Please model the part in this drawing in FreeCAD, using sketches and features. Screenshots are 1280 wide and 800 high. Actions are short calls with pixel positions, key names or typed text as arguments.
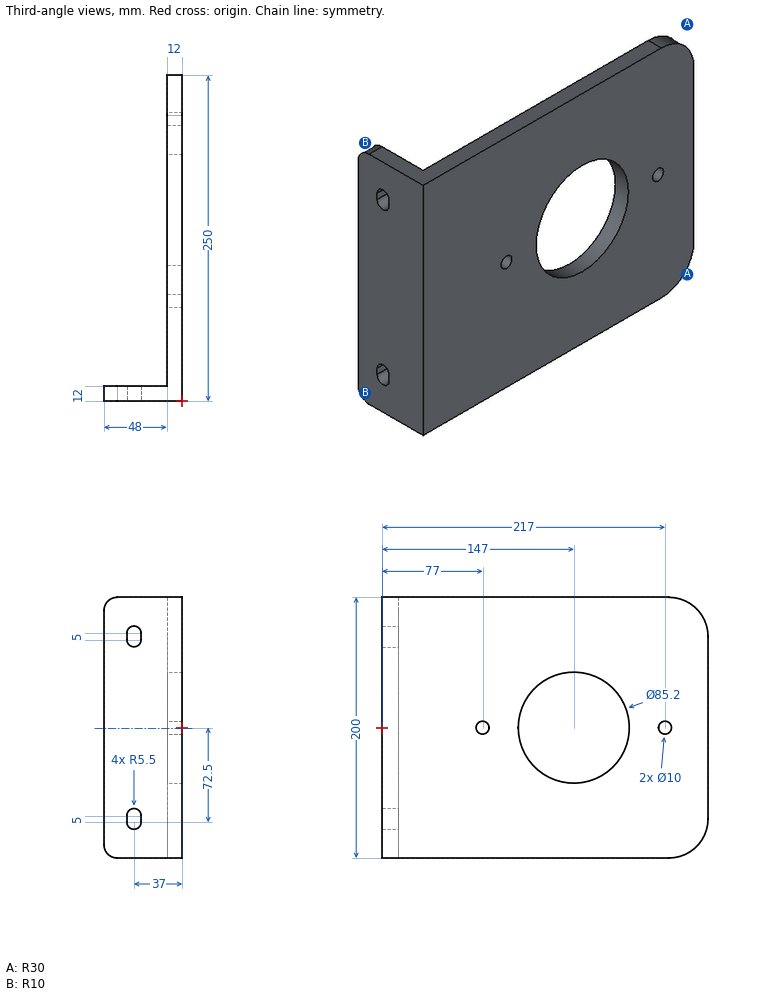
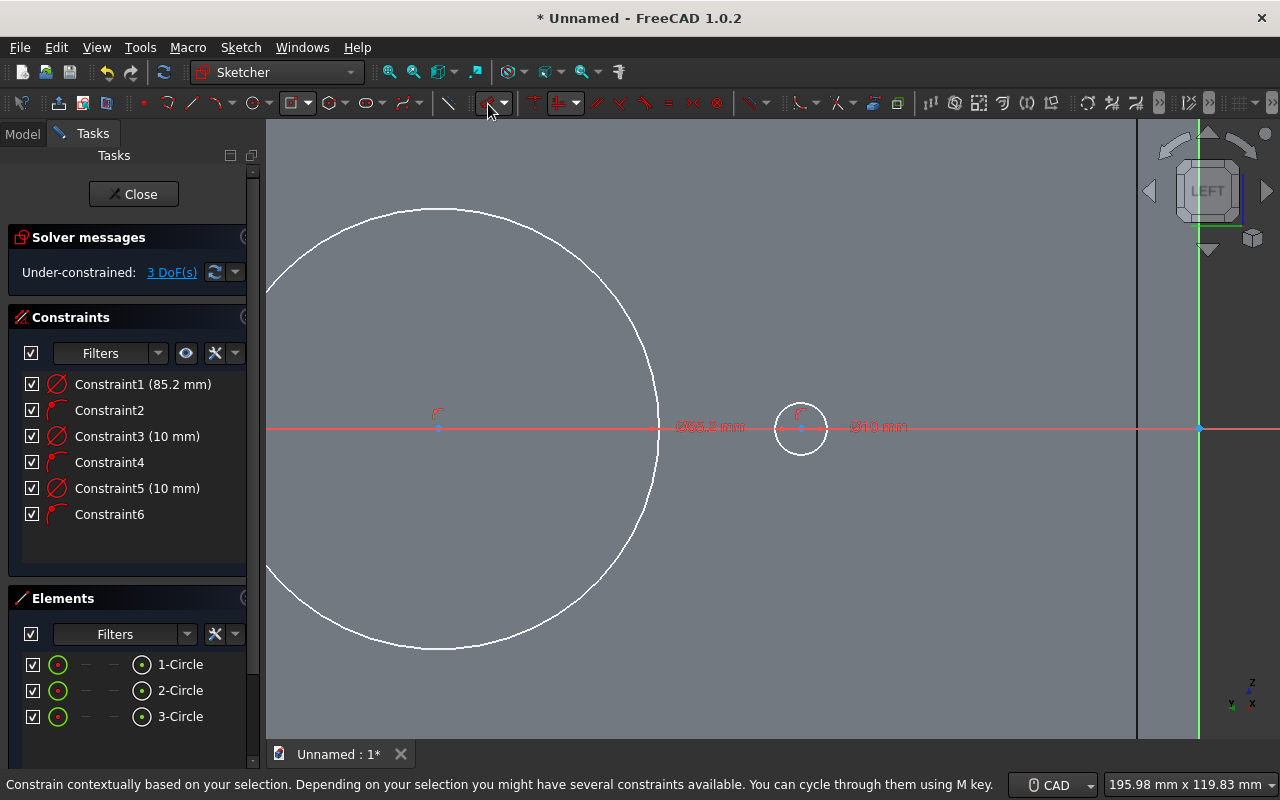
click(801, 429)
click(958, 463)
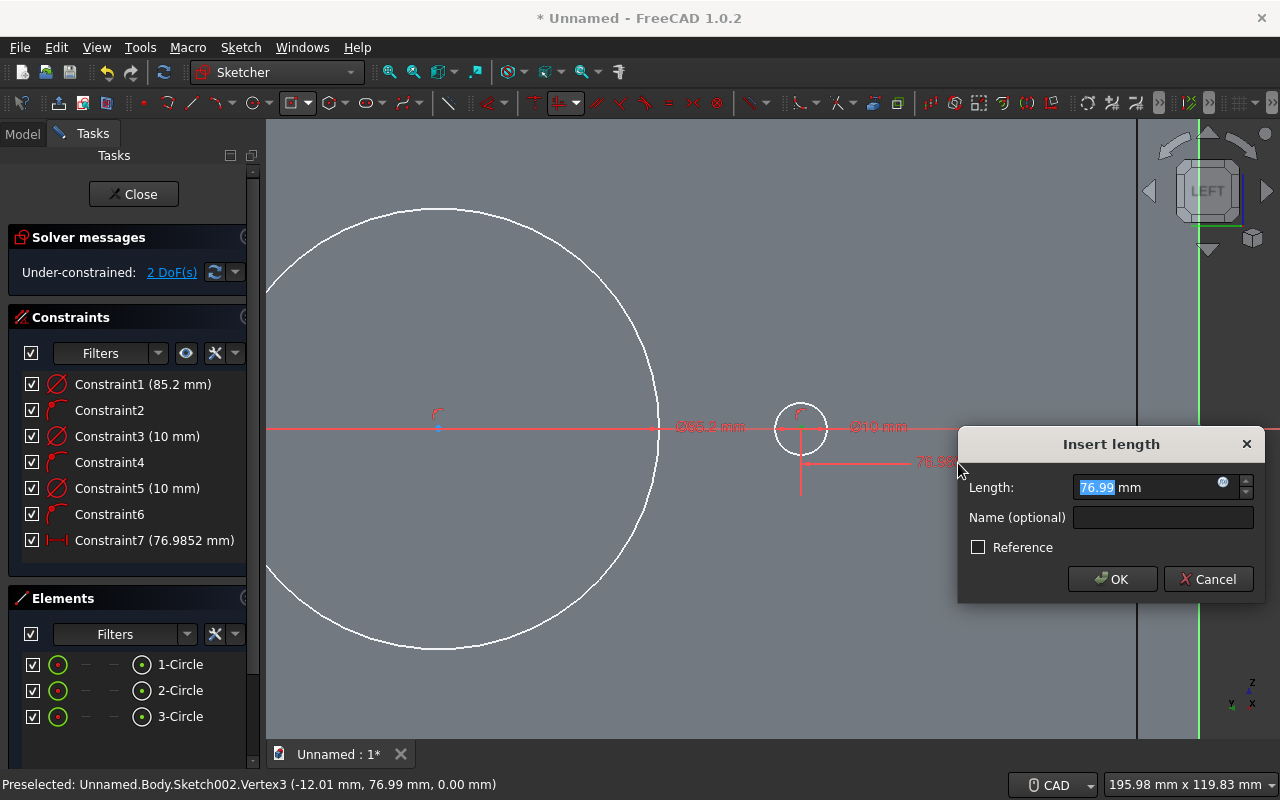
text(77)
key(Return)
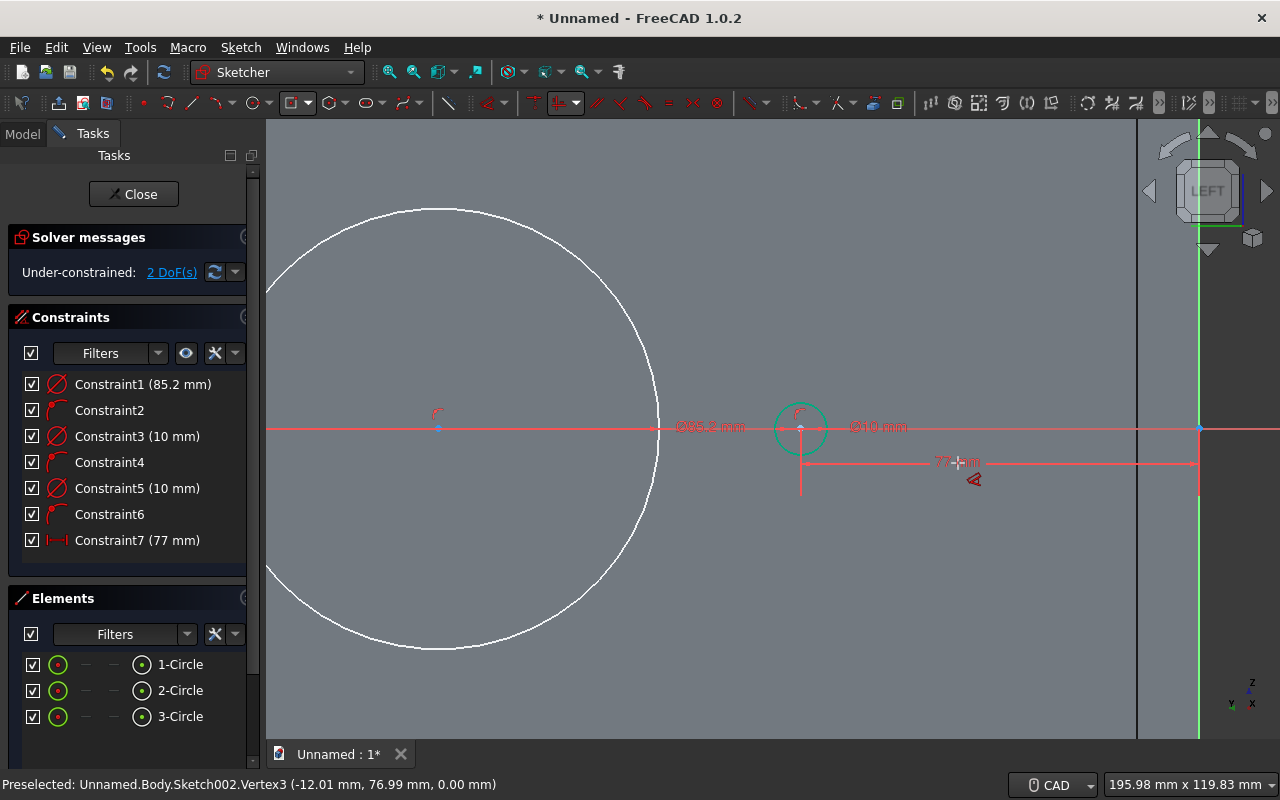
click(439, 429)
click(777, 463)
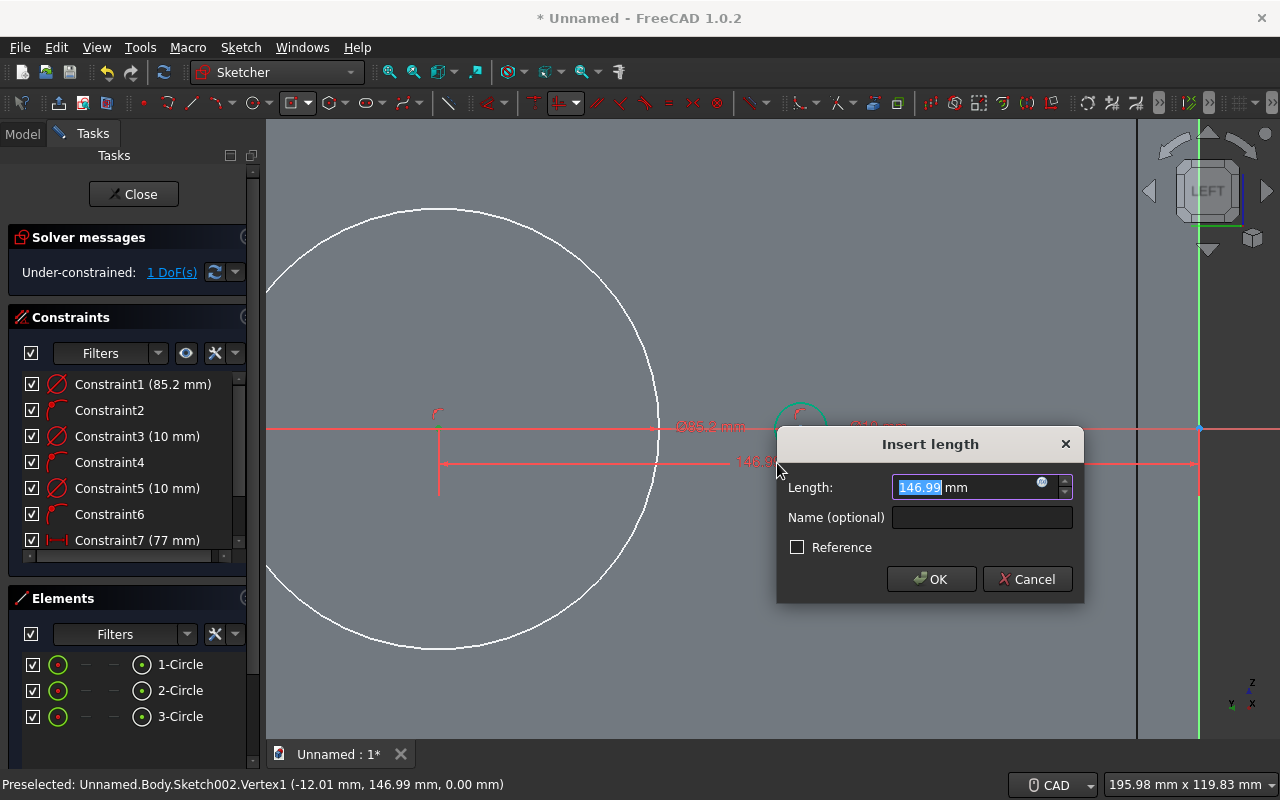
text(147)
key(Return)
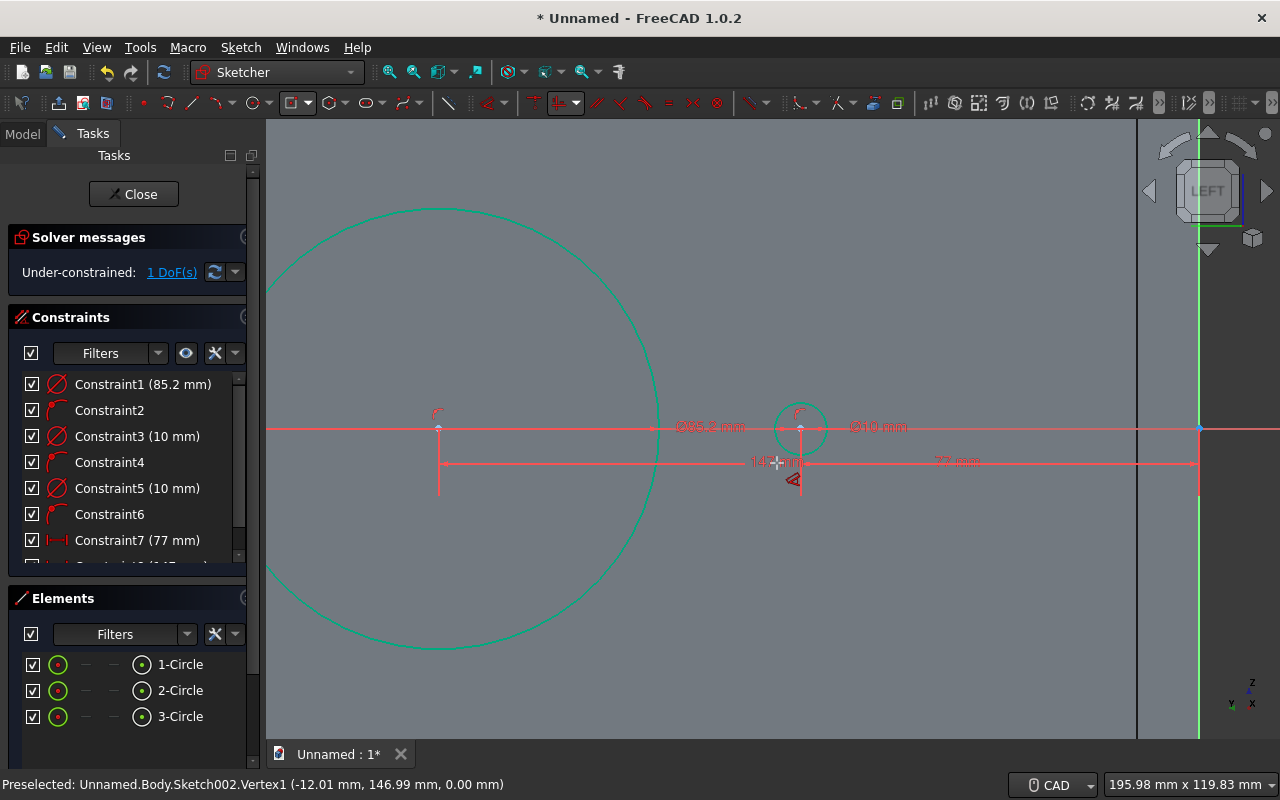
scroll(801, 429, down, 3)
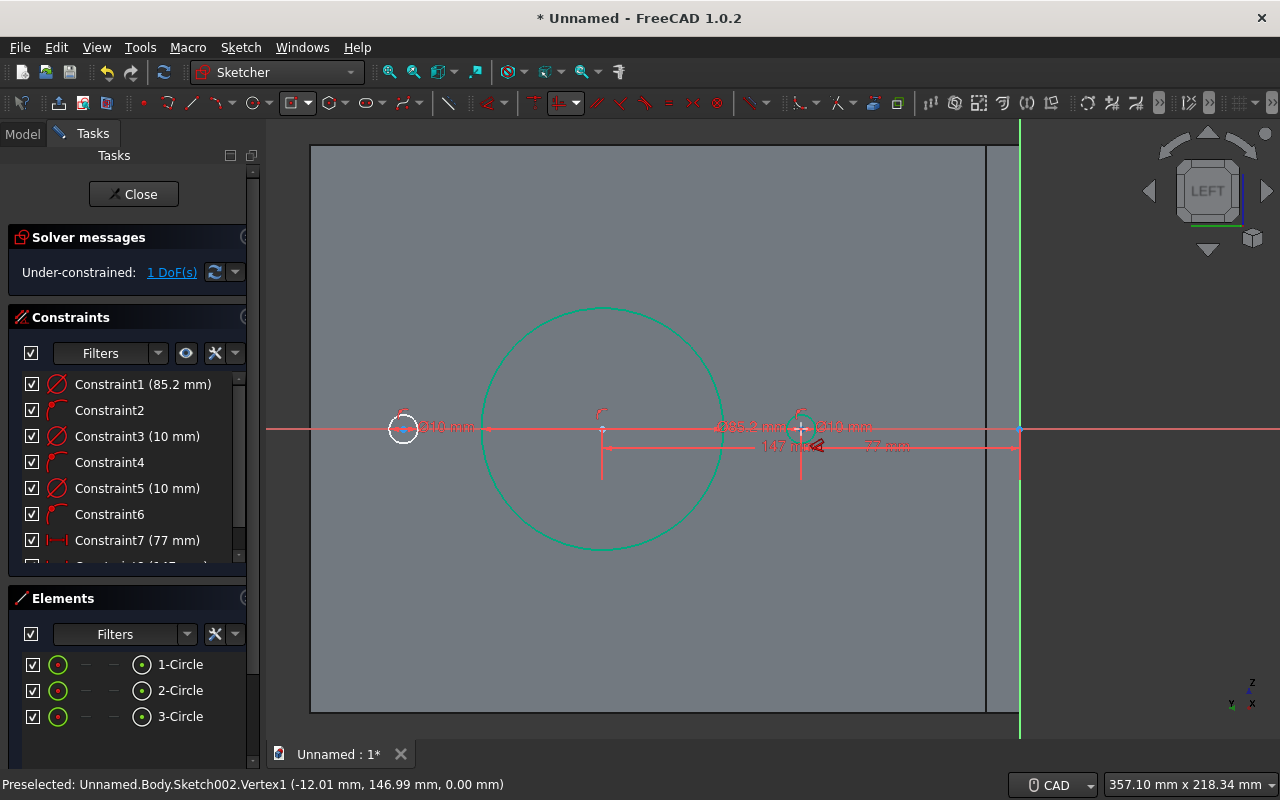
click(404, 429)
click(570, 463)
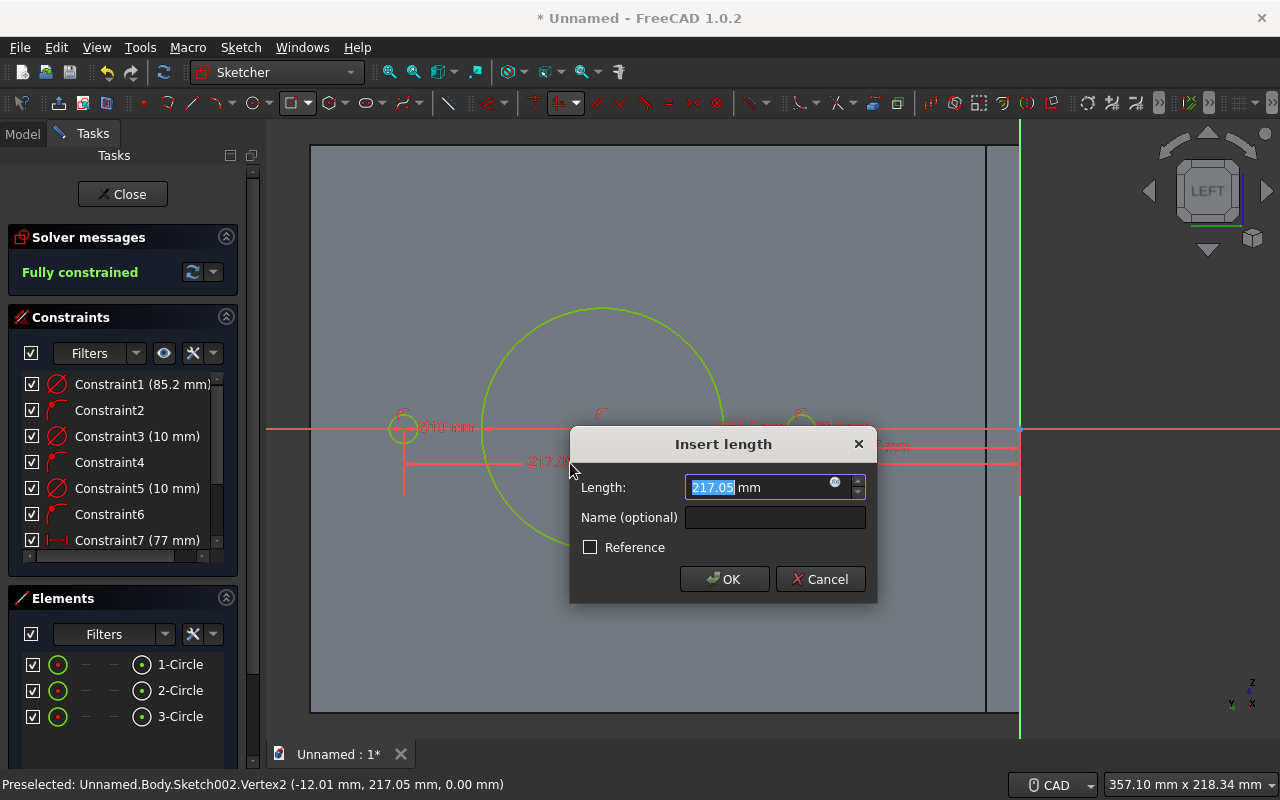
text(217)
key(Return)
key(Escape)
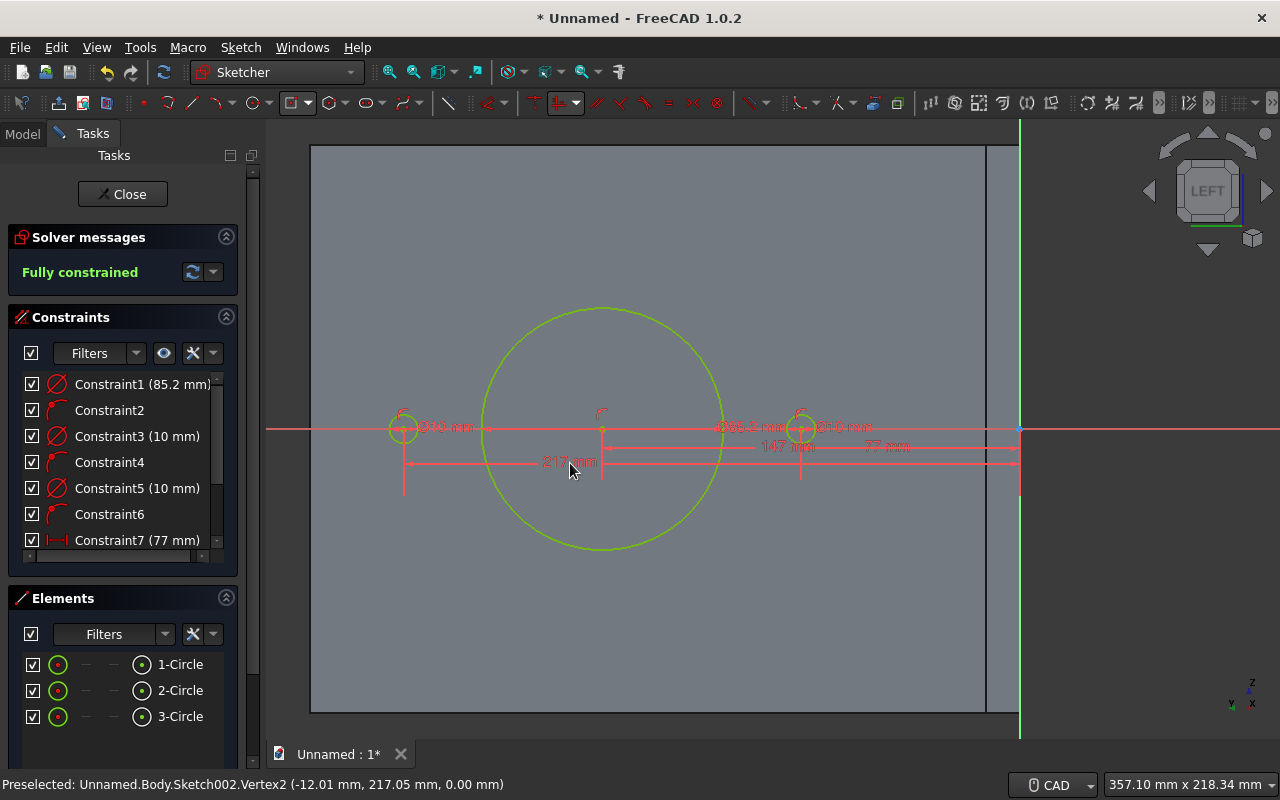
click(123, 194)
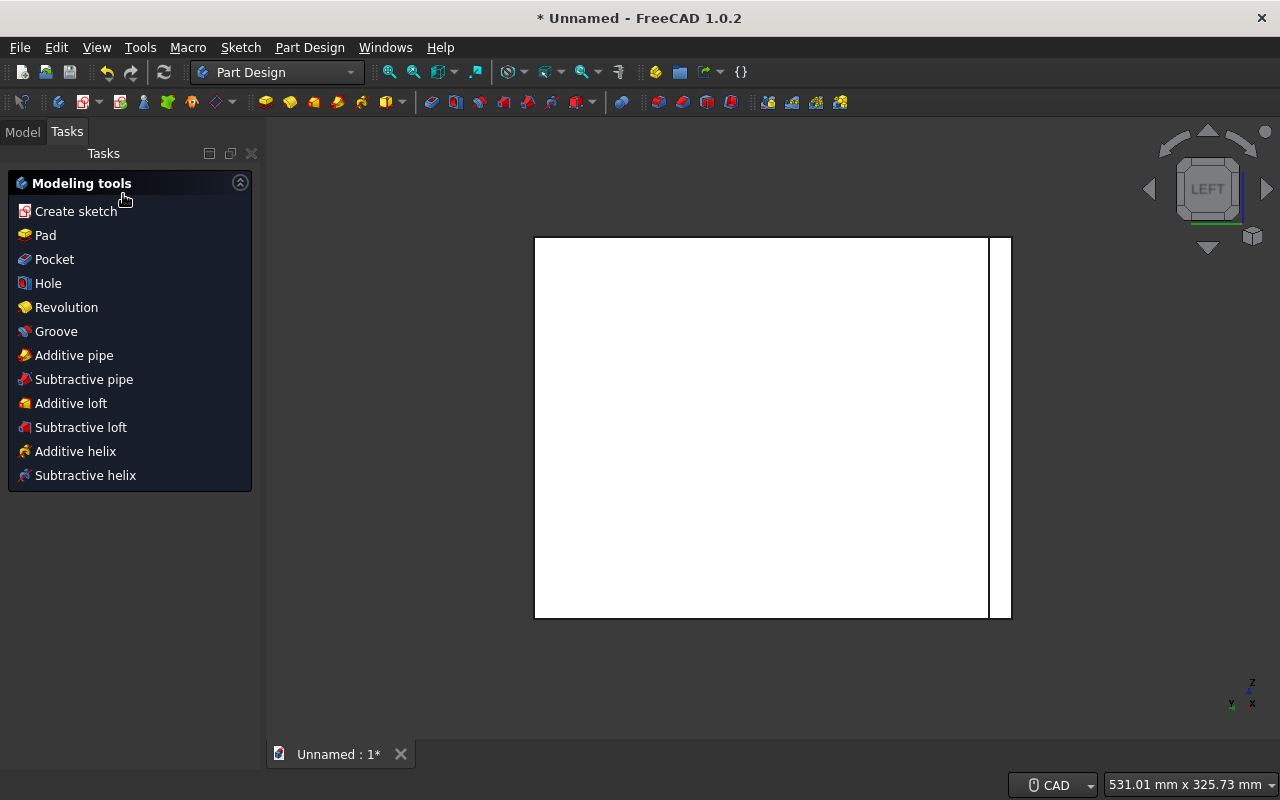
click(432, 102)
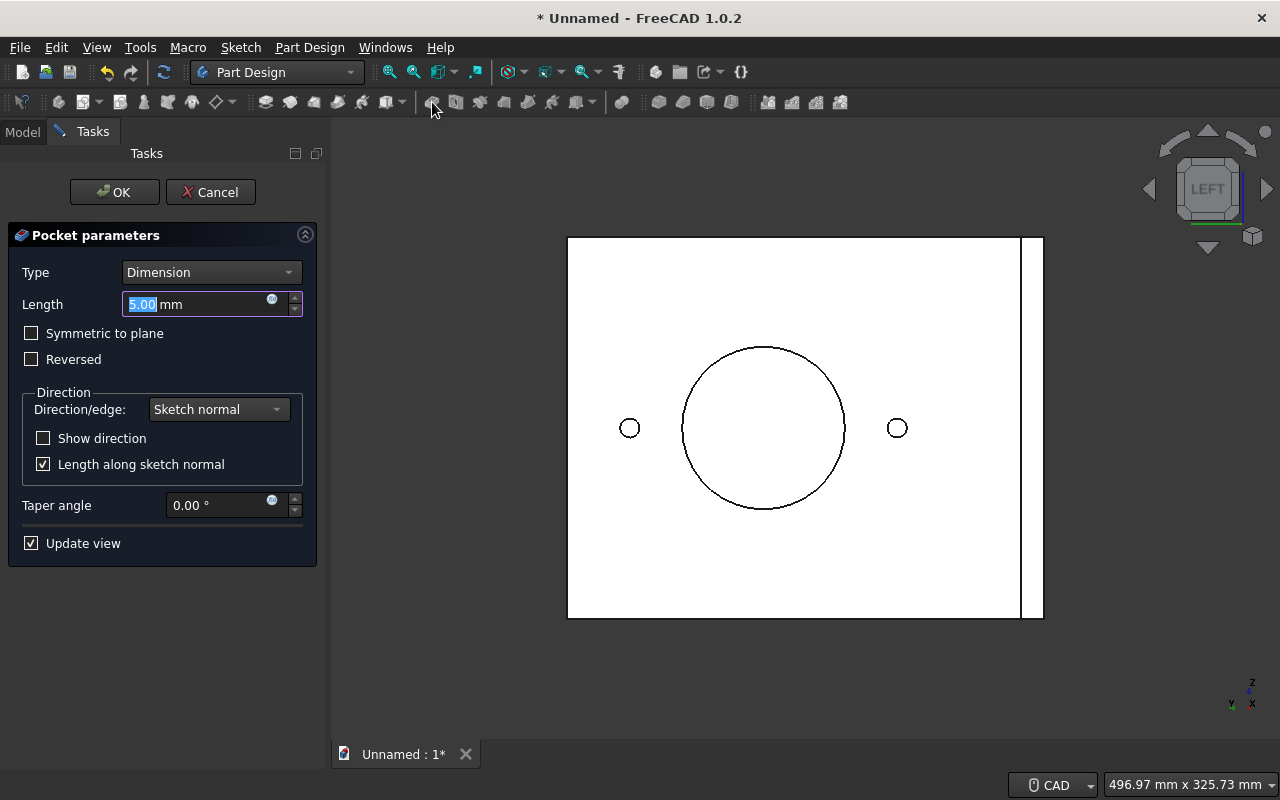
click(212, 272)